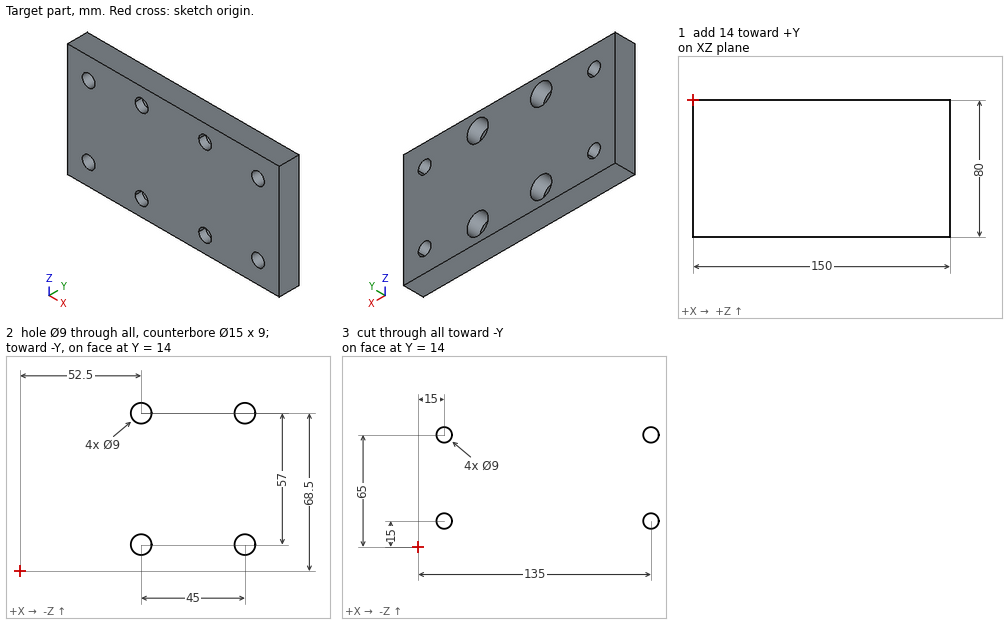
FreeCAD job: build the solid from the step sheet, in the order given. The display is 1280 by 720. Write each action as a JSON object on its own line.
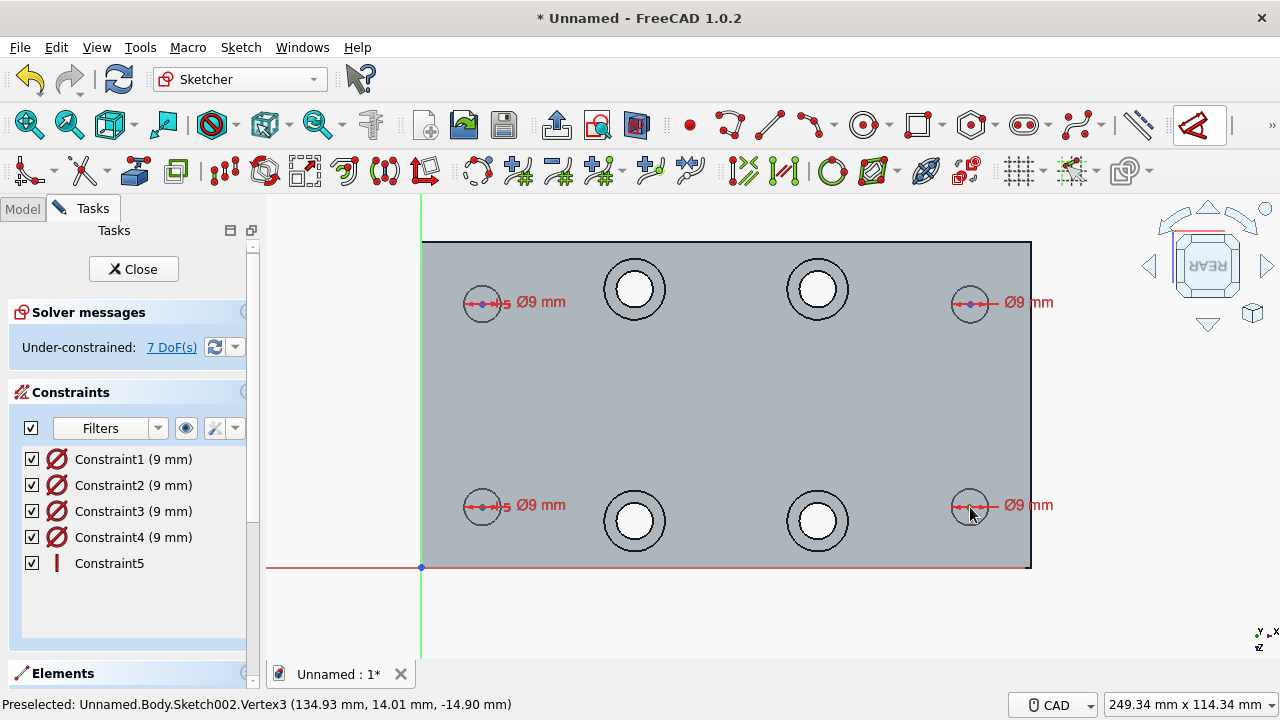
{"action": "key", "text": "h"}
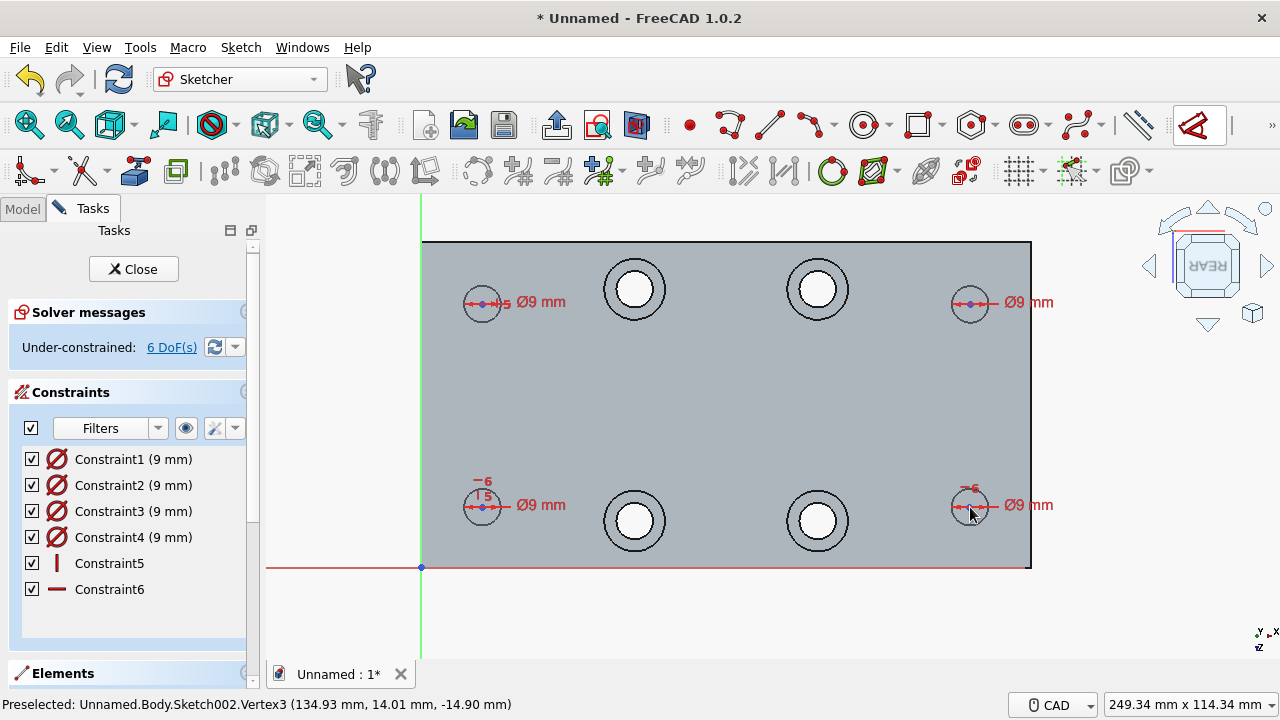
{"action": "left_click", "coordinate": [970, 507]}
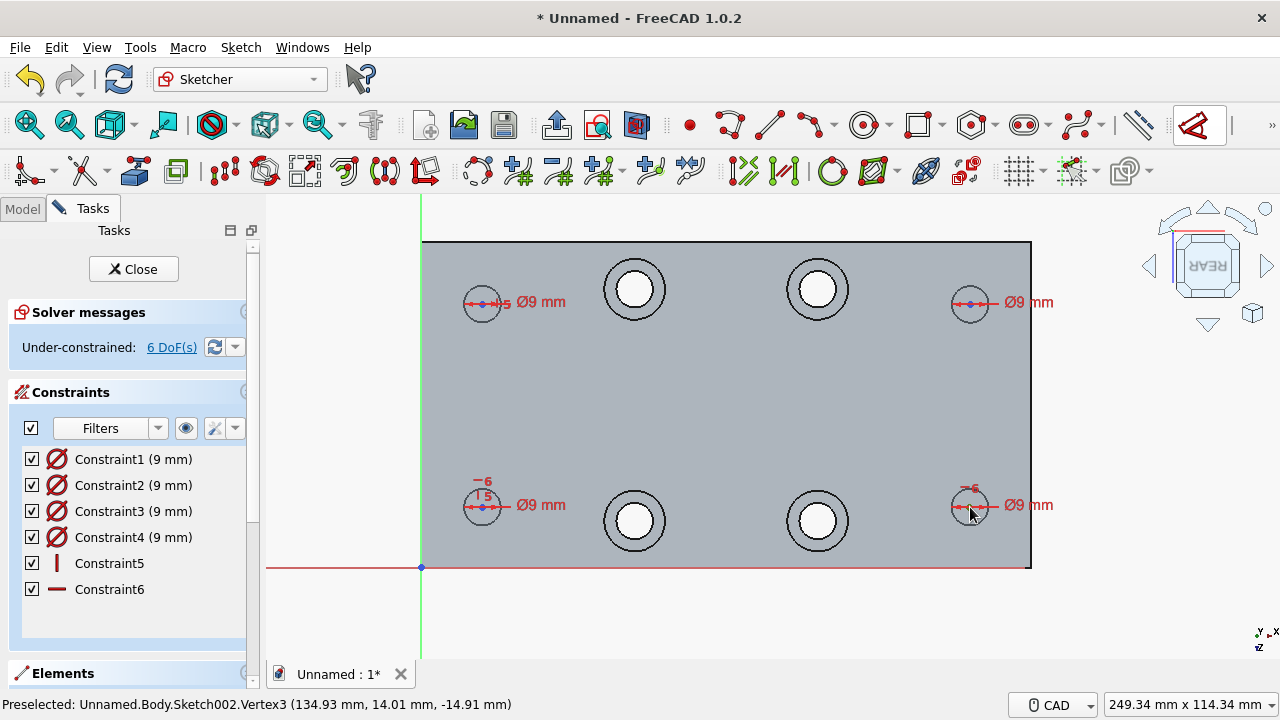
{"action": "left_click", "coordinate": [970, 304]}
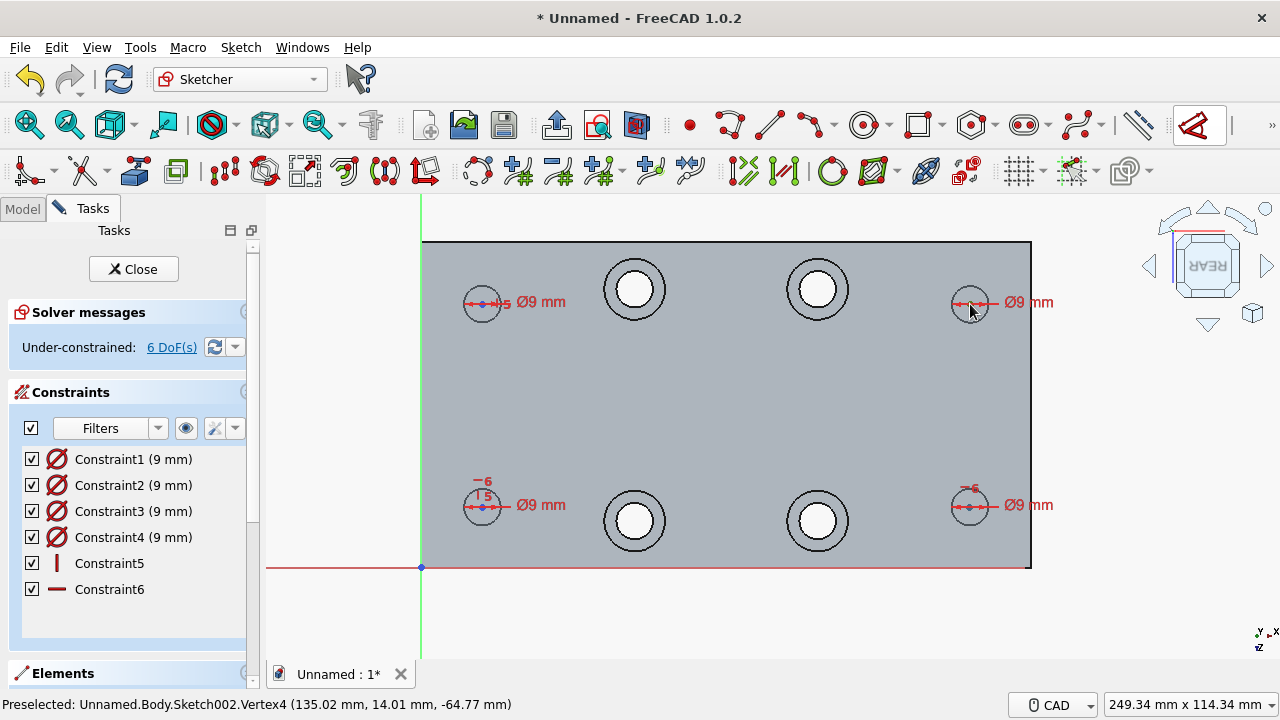
{"action": "key", "text": "v"}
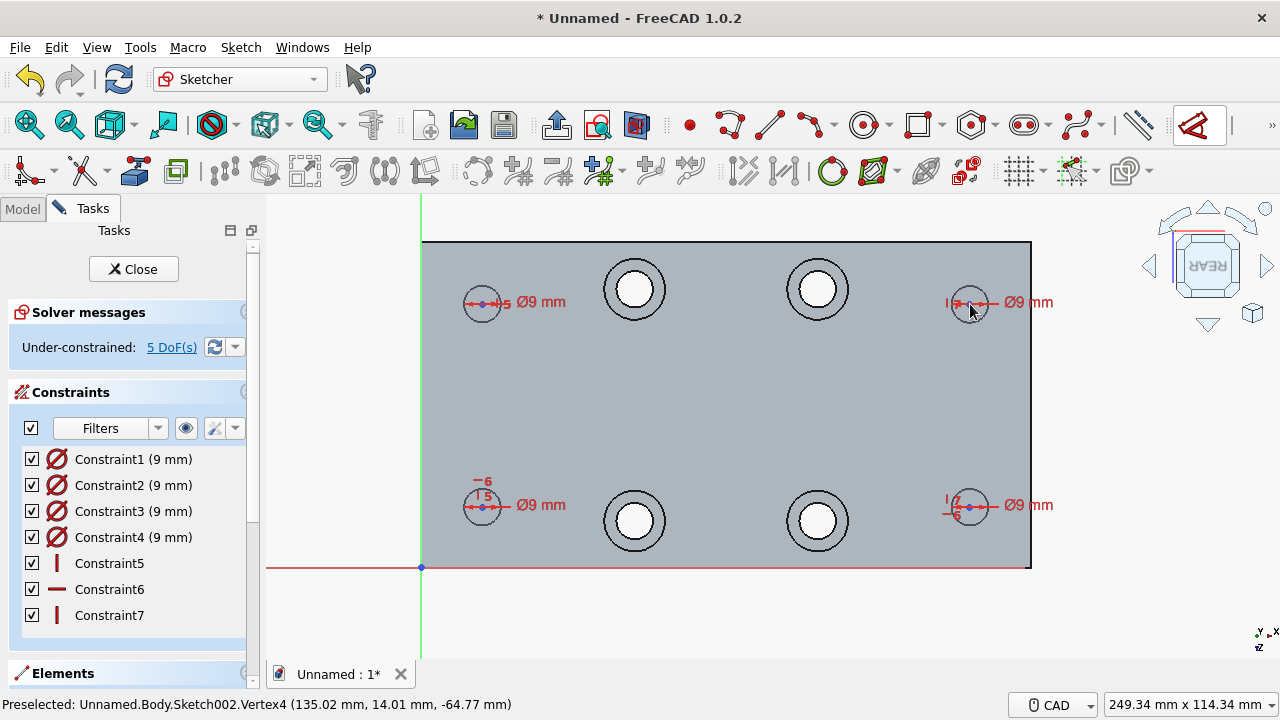
{"action": "left_click", "coordinate": [482, 304]}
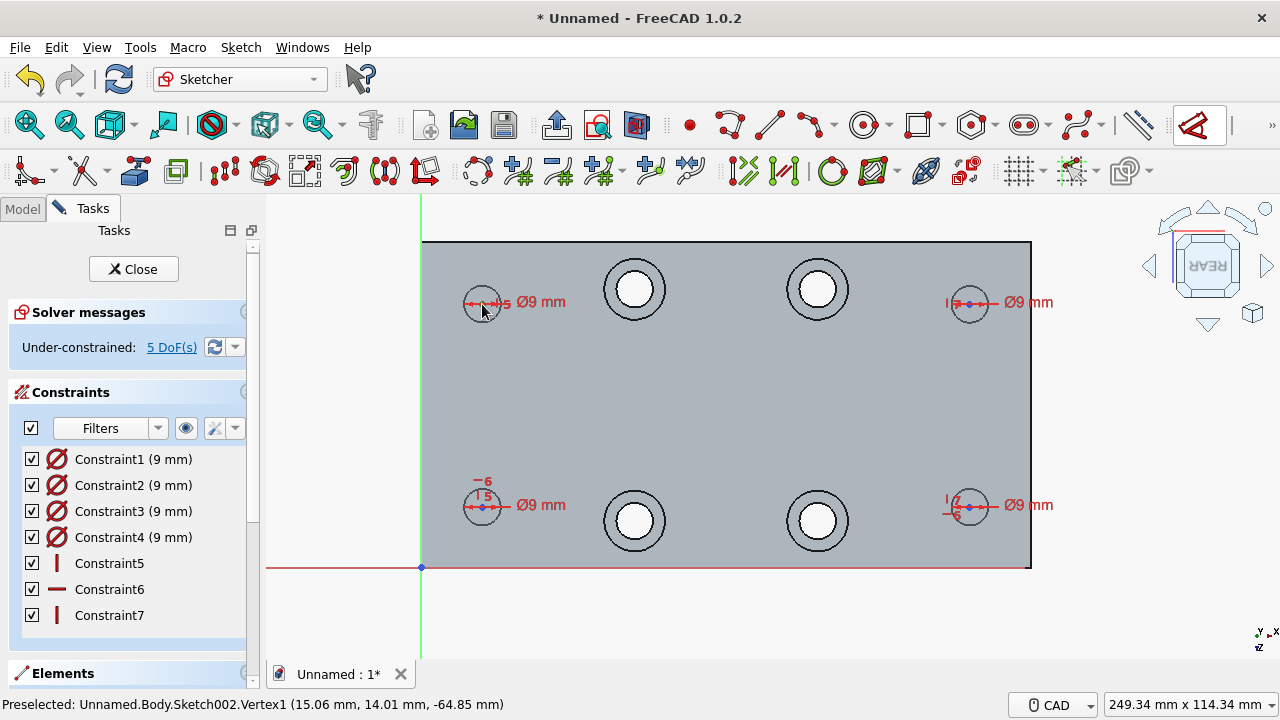
{"action": "left_click", "coordinate": [970, 304]}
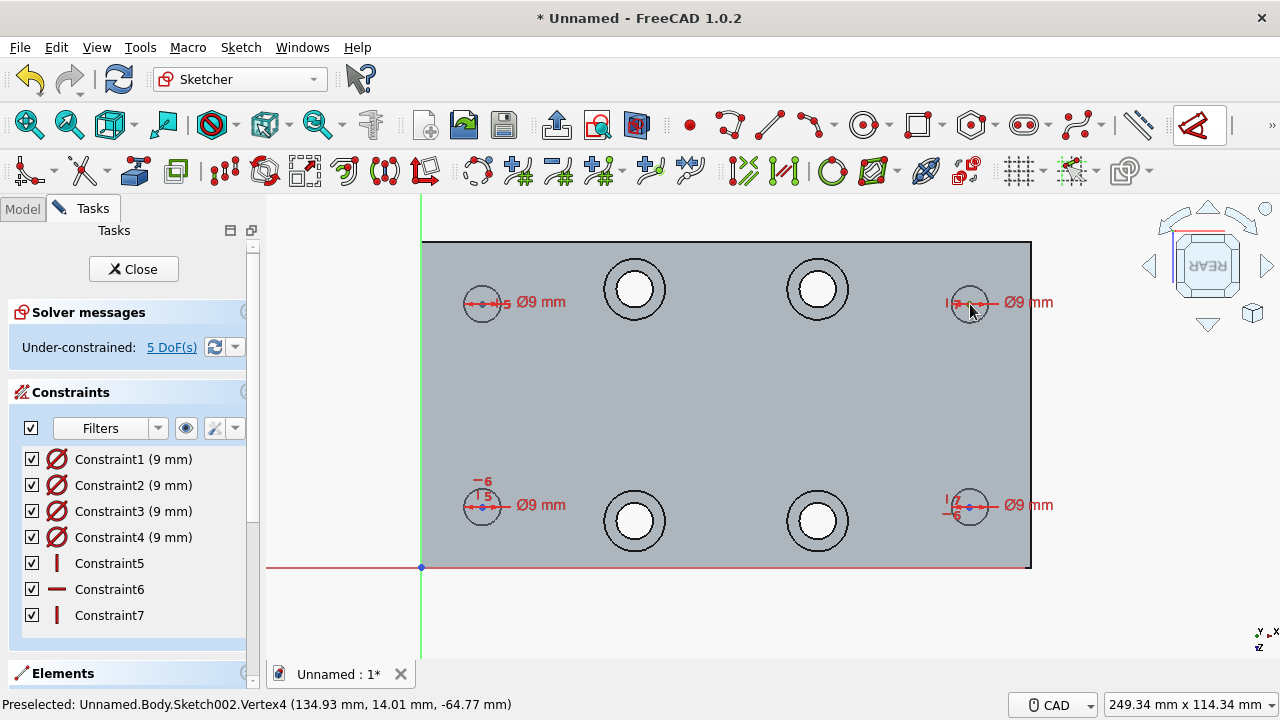
{"action": "key", "text": "h"}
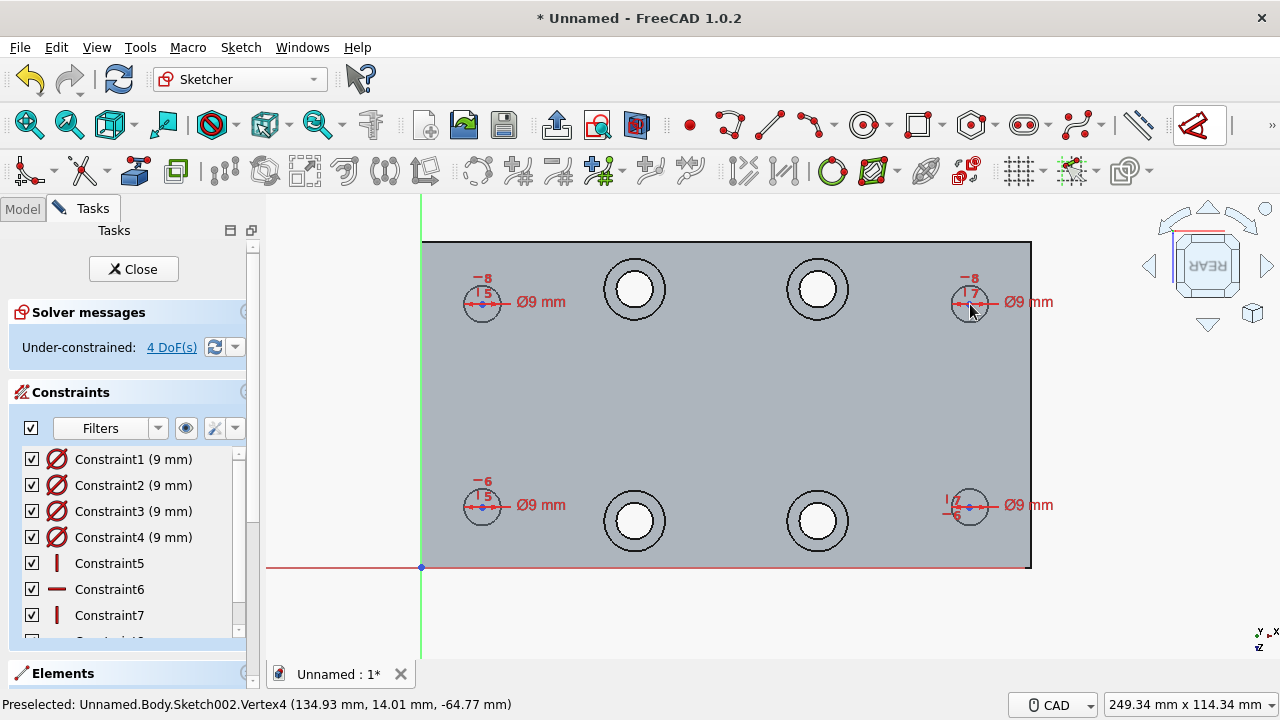
{"action": "left_click", "coordinate": [482, 304]}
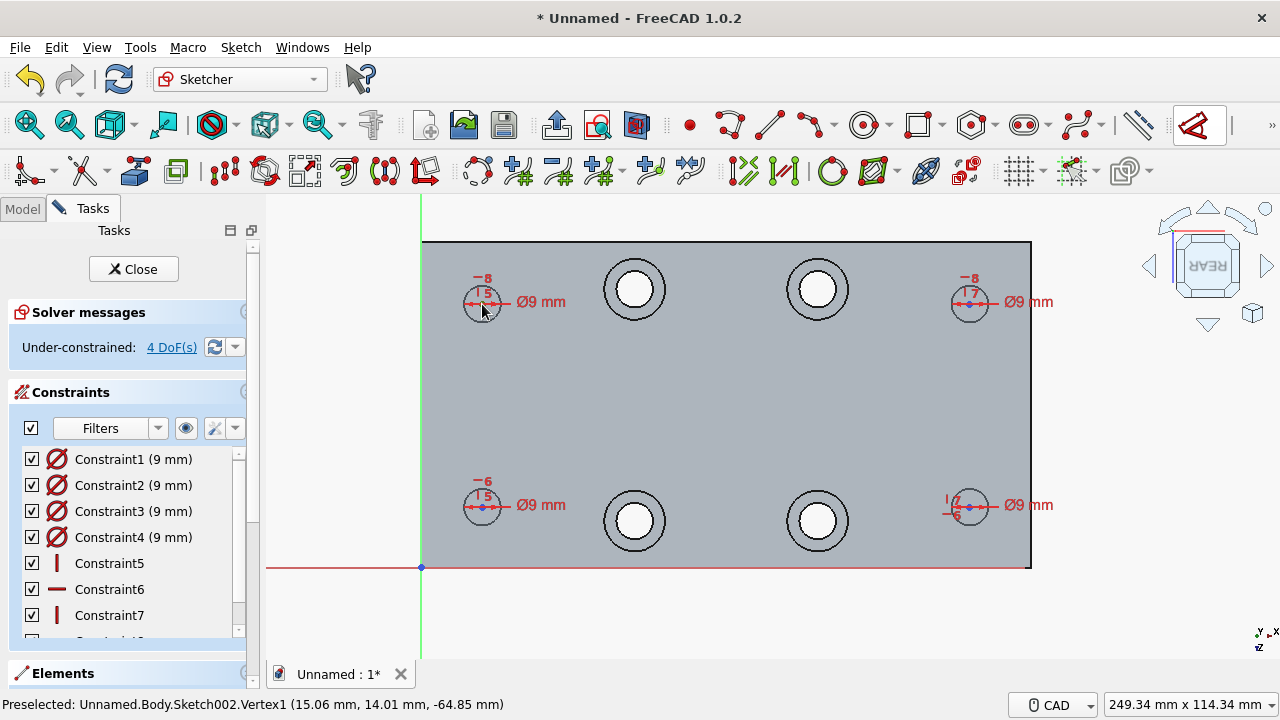
{"action": "left_click", "coordinate": [1220, 126]}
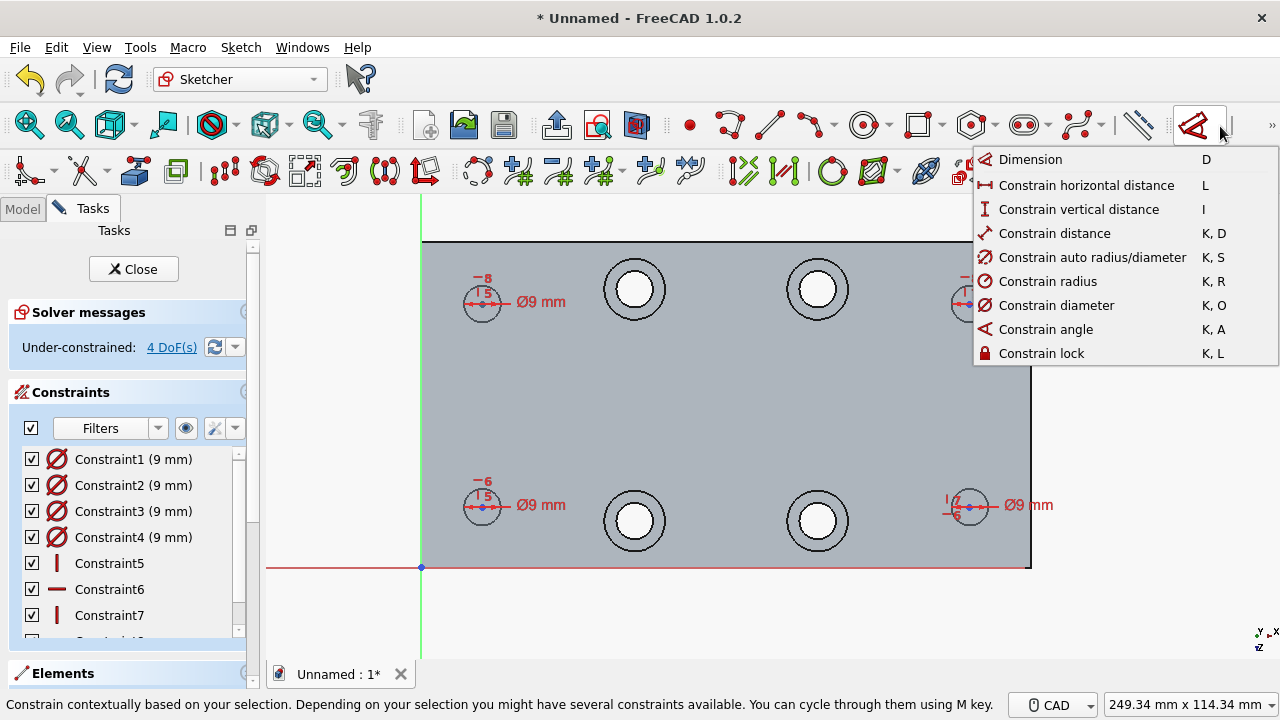
{"action": "left_click", "coordinate": [1126, 185]}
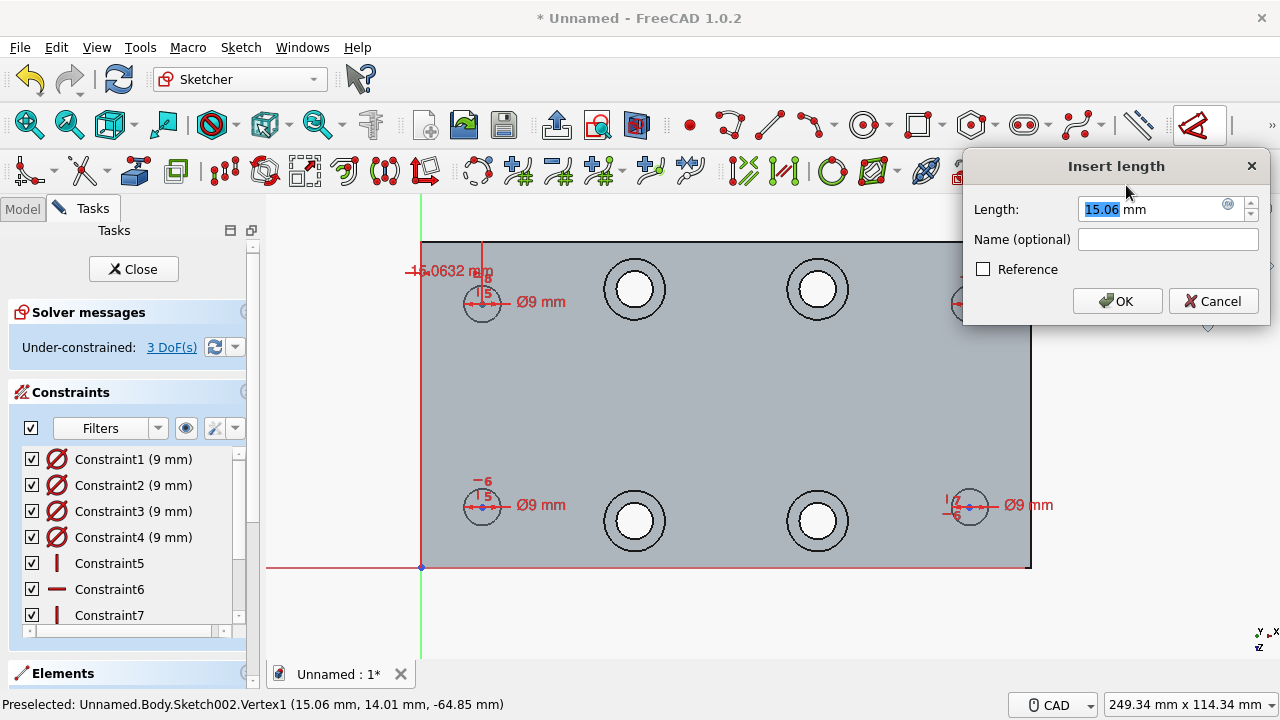
{"action": "type", "text": "15"}
{"action": "key", "text": "Return"}